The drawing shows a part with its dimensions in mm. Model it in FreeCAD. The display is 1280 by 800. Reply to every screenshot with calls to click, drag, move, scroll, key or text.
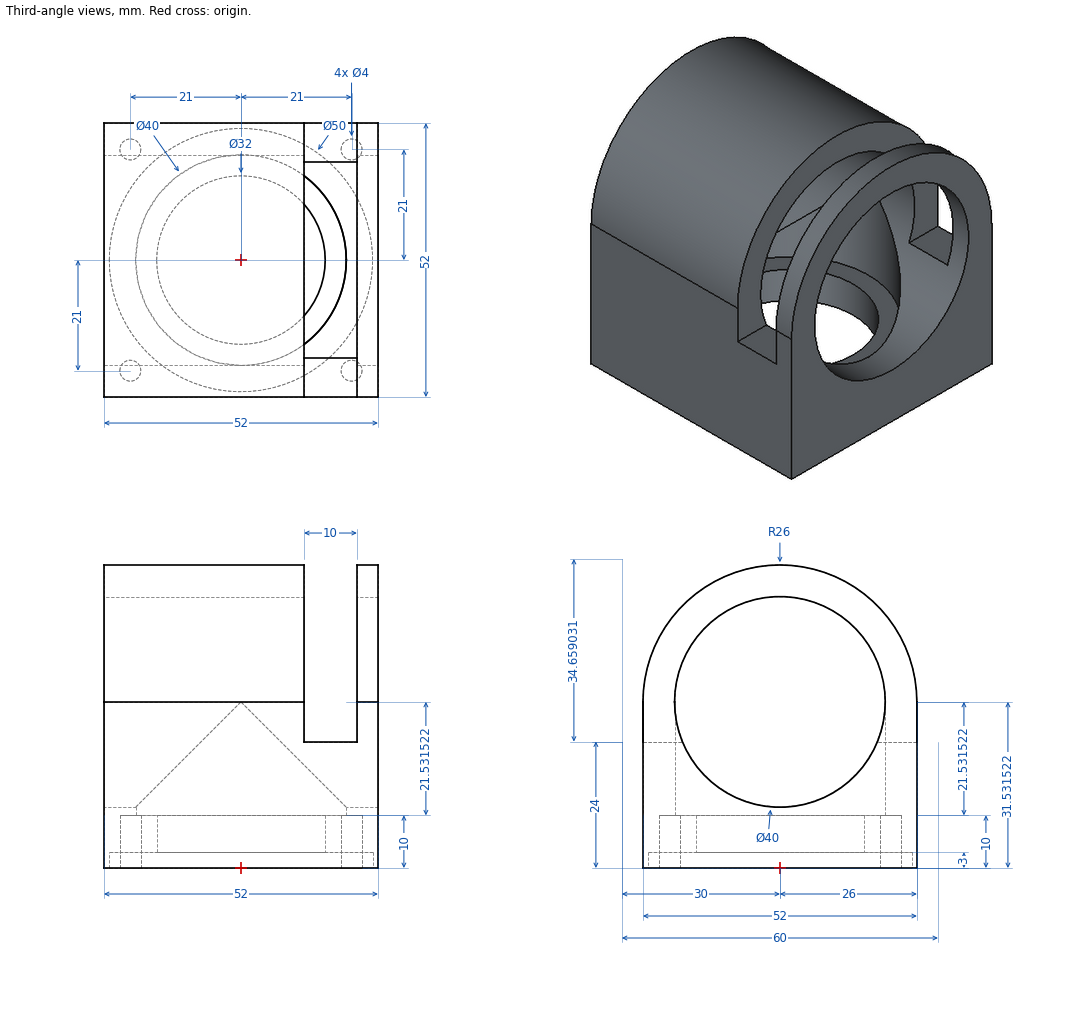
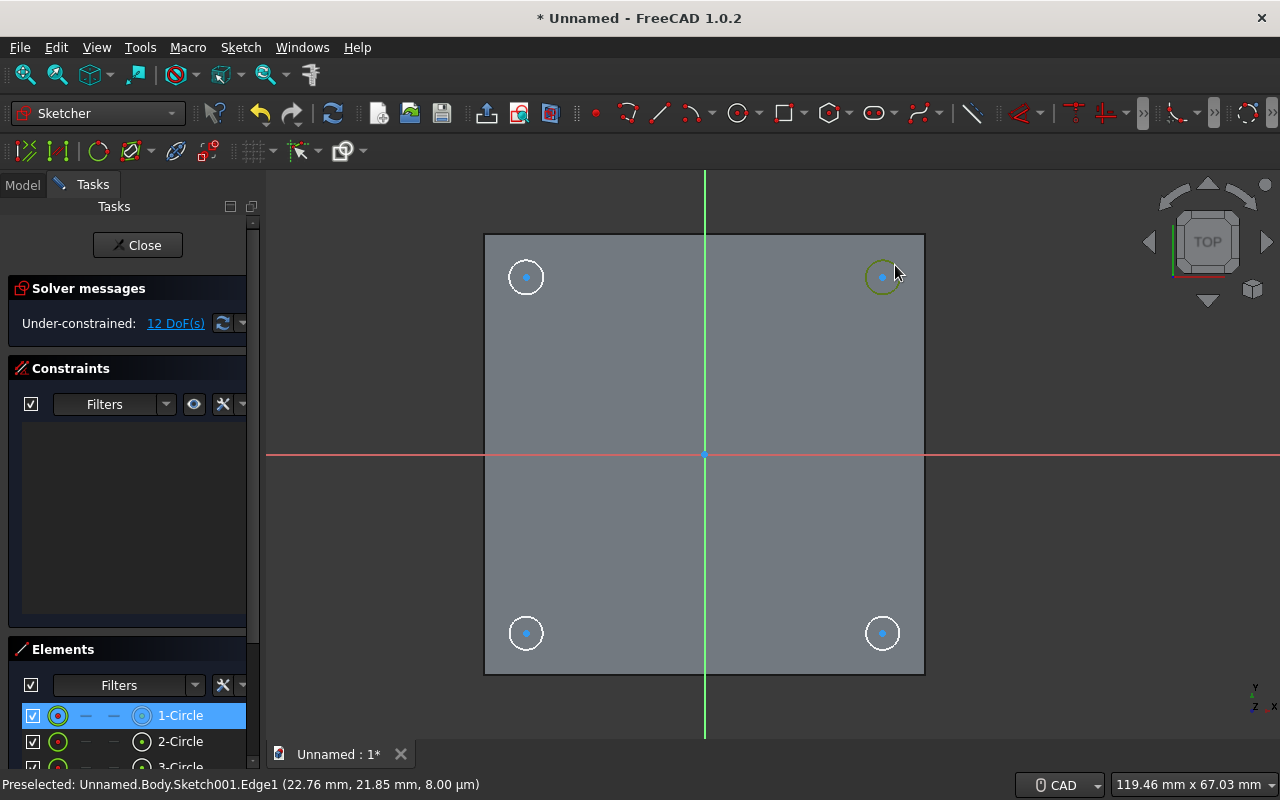
click(538, 265)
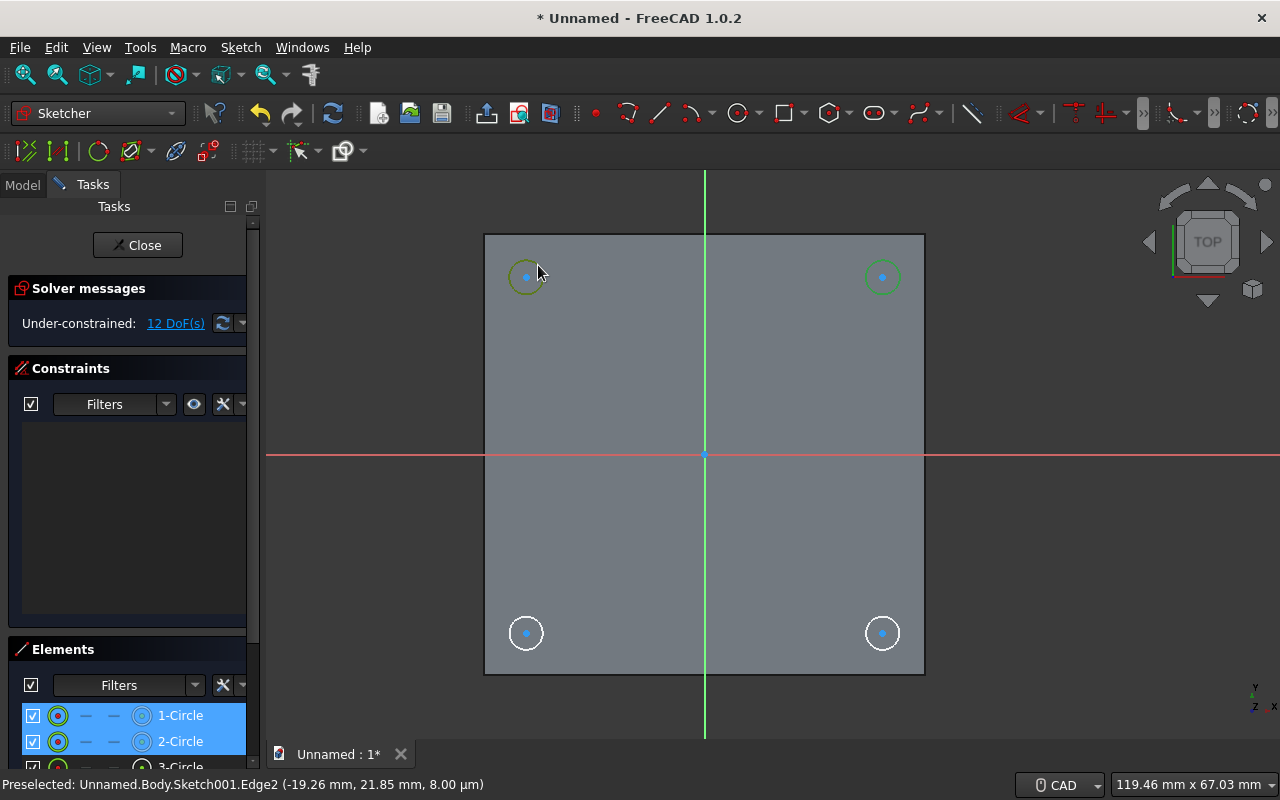
click(538, 621)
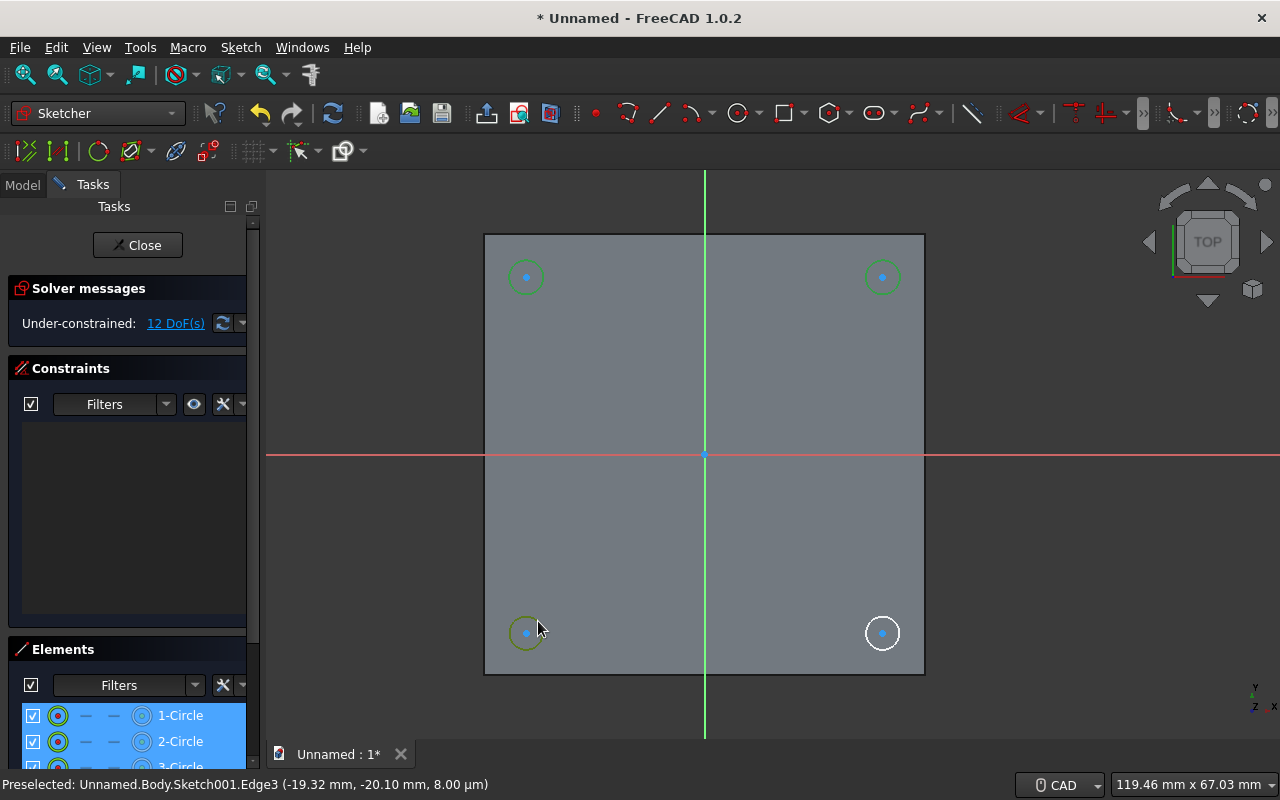
click(894, 621)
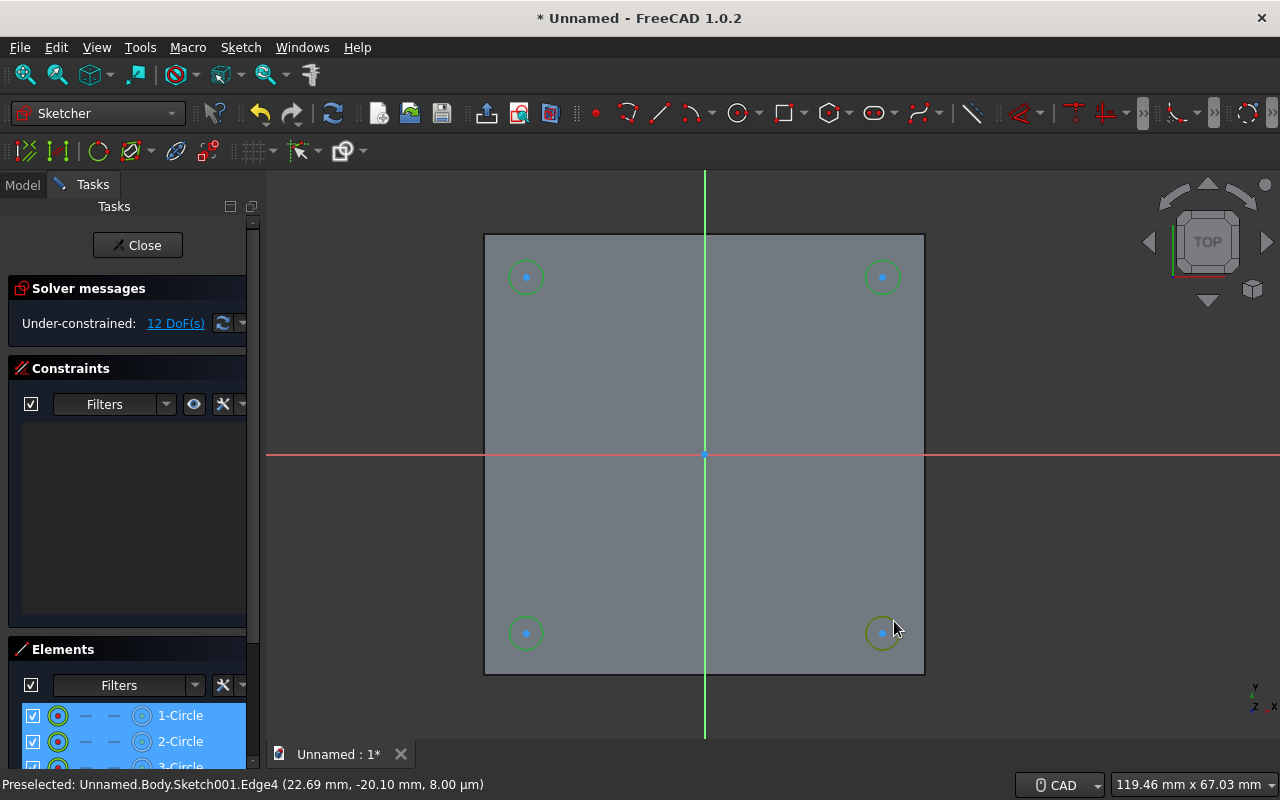
key(e)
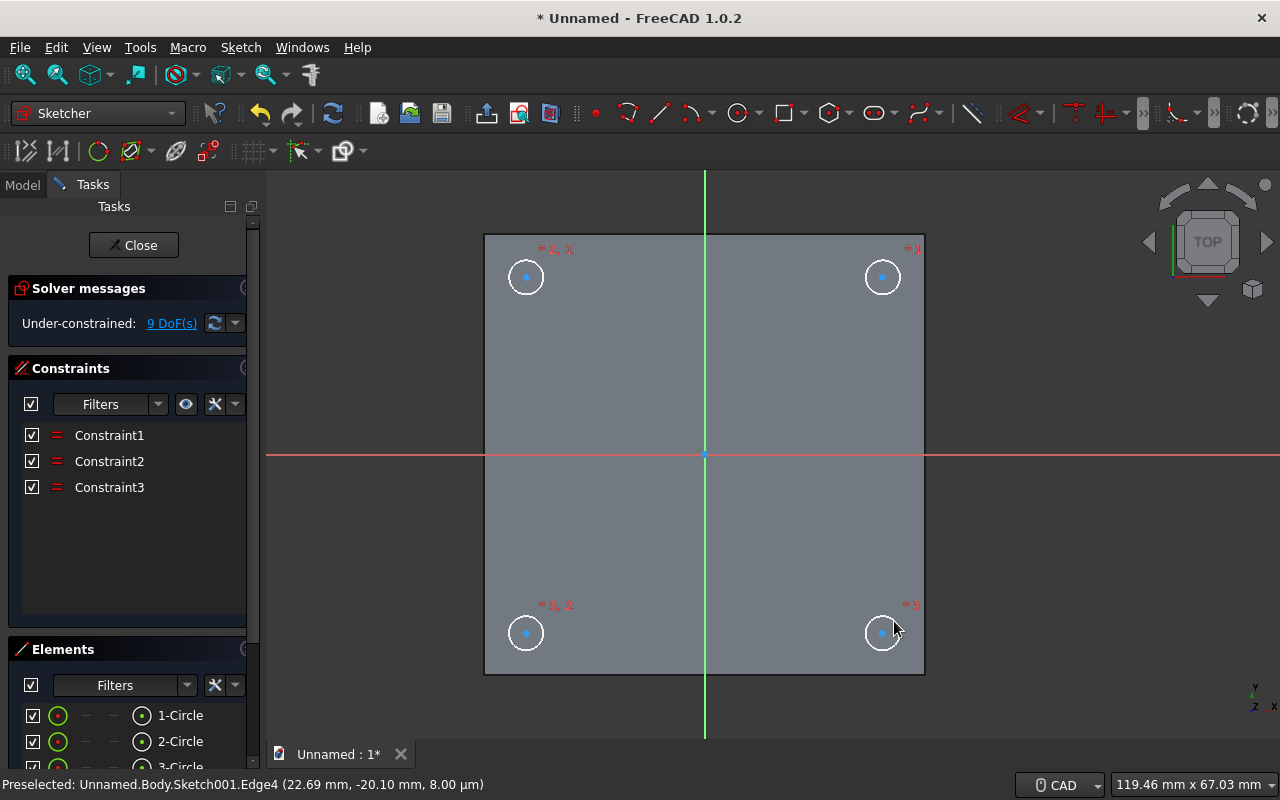
click(883, 277)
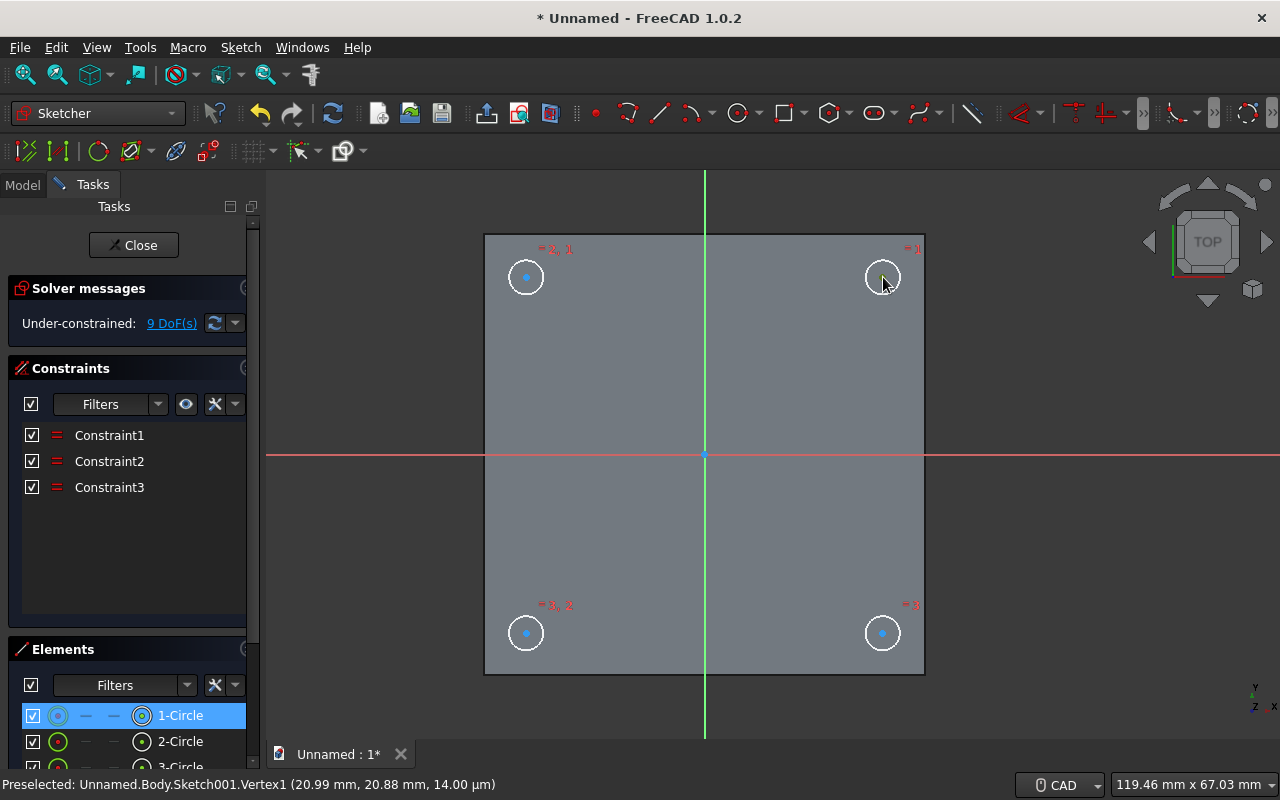
click(526, 277)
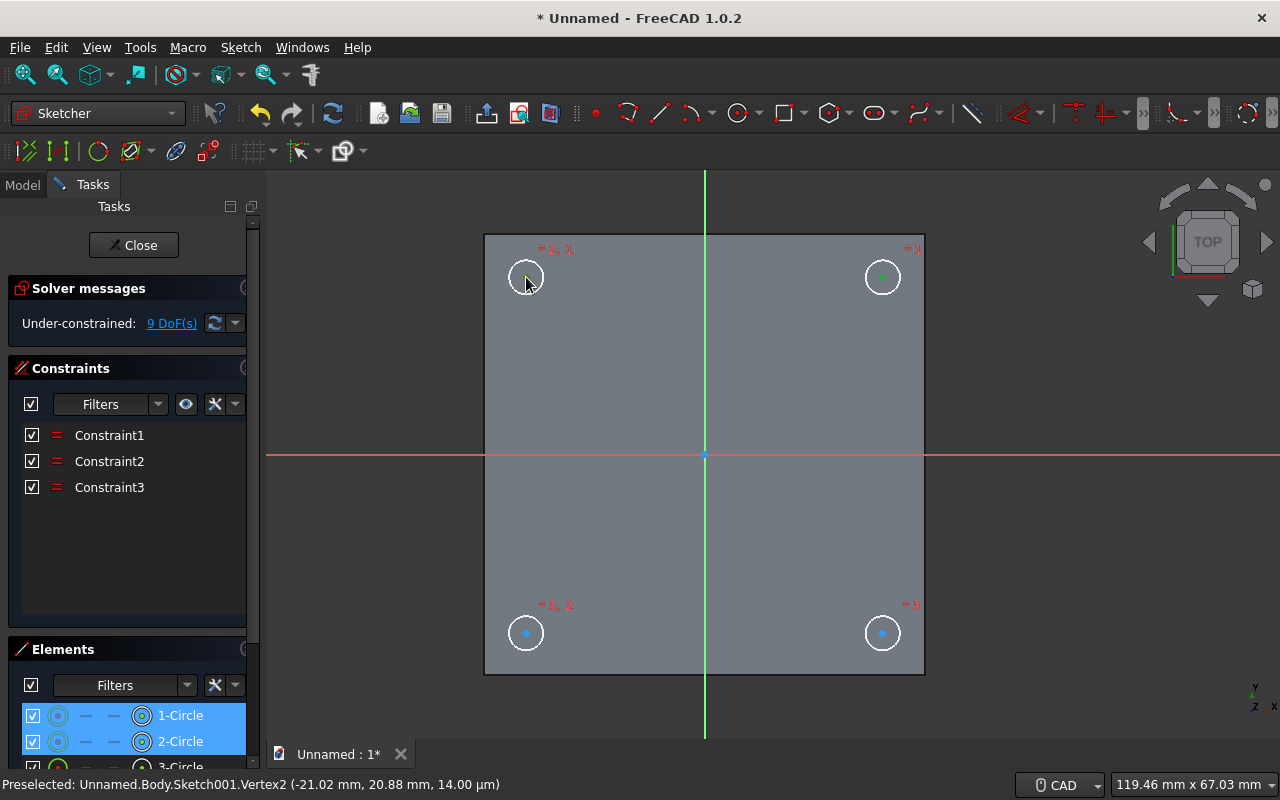
click(1128, 114)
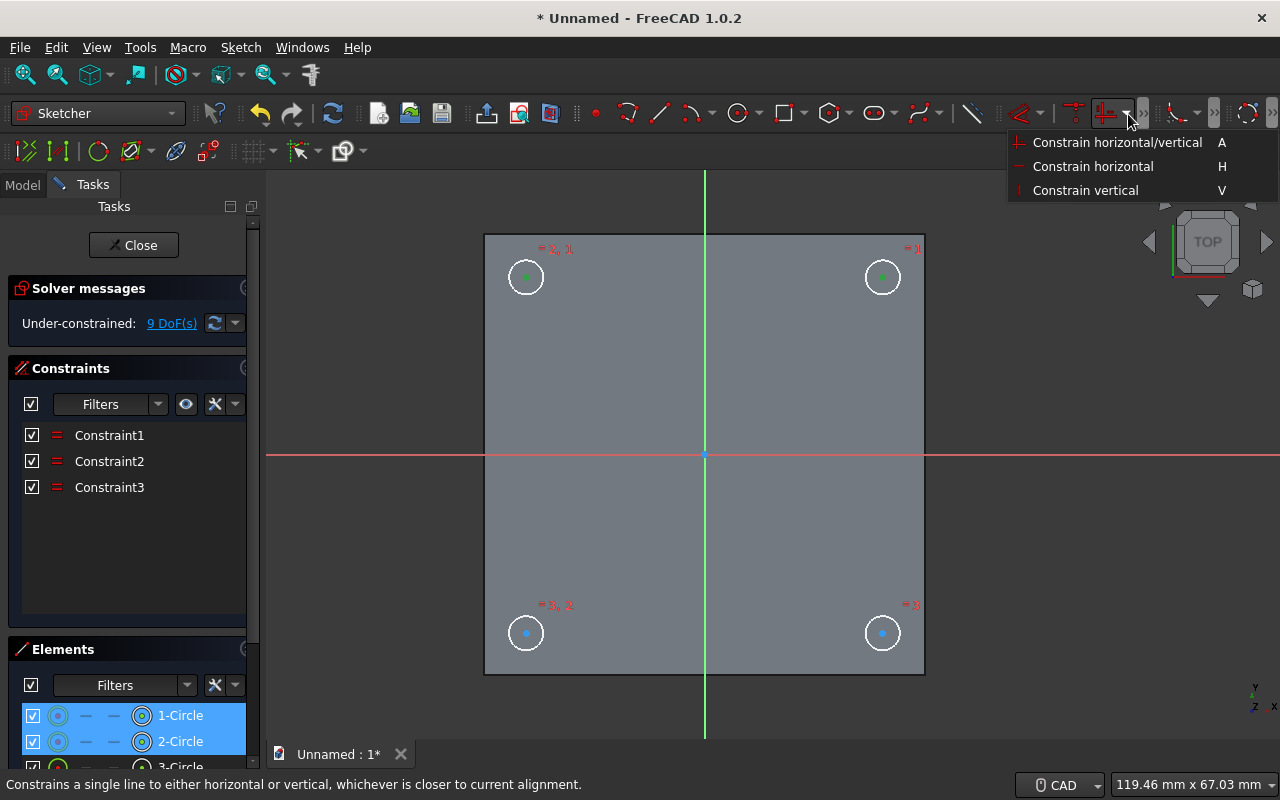
click(1143, 166)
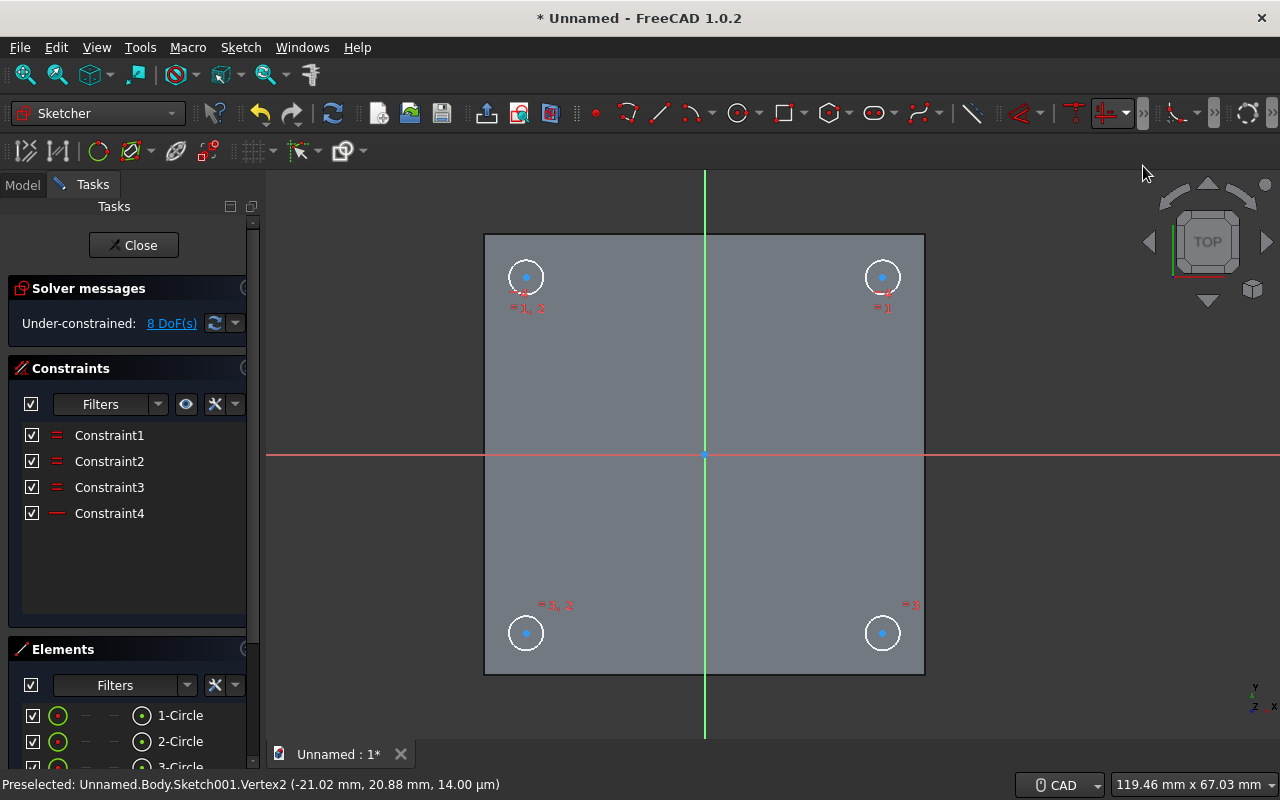
click(526, 277)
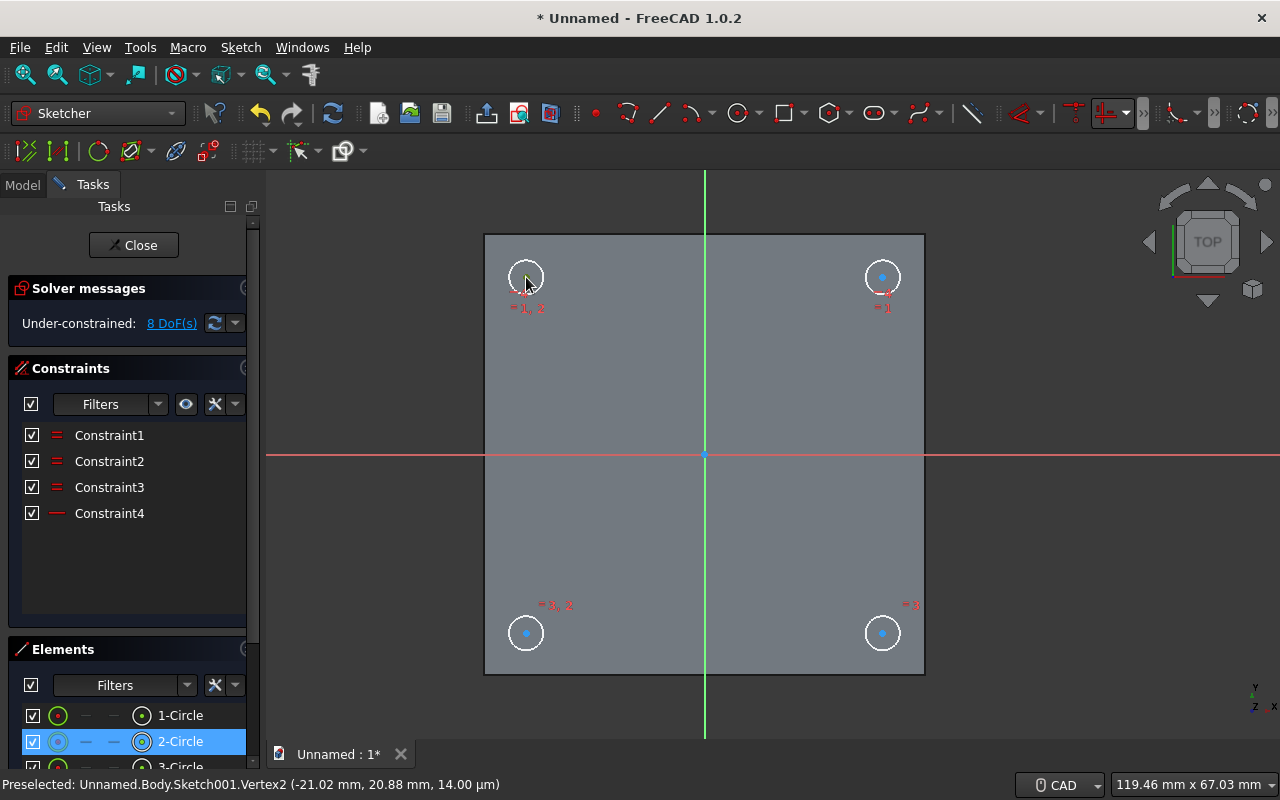
click(526, 633)